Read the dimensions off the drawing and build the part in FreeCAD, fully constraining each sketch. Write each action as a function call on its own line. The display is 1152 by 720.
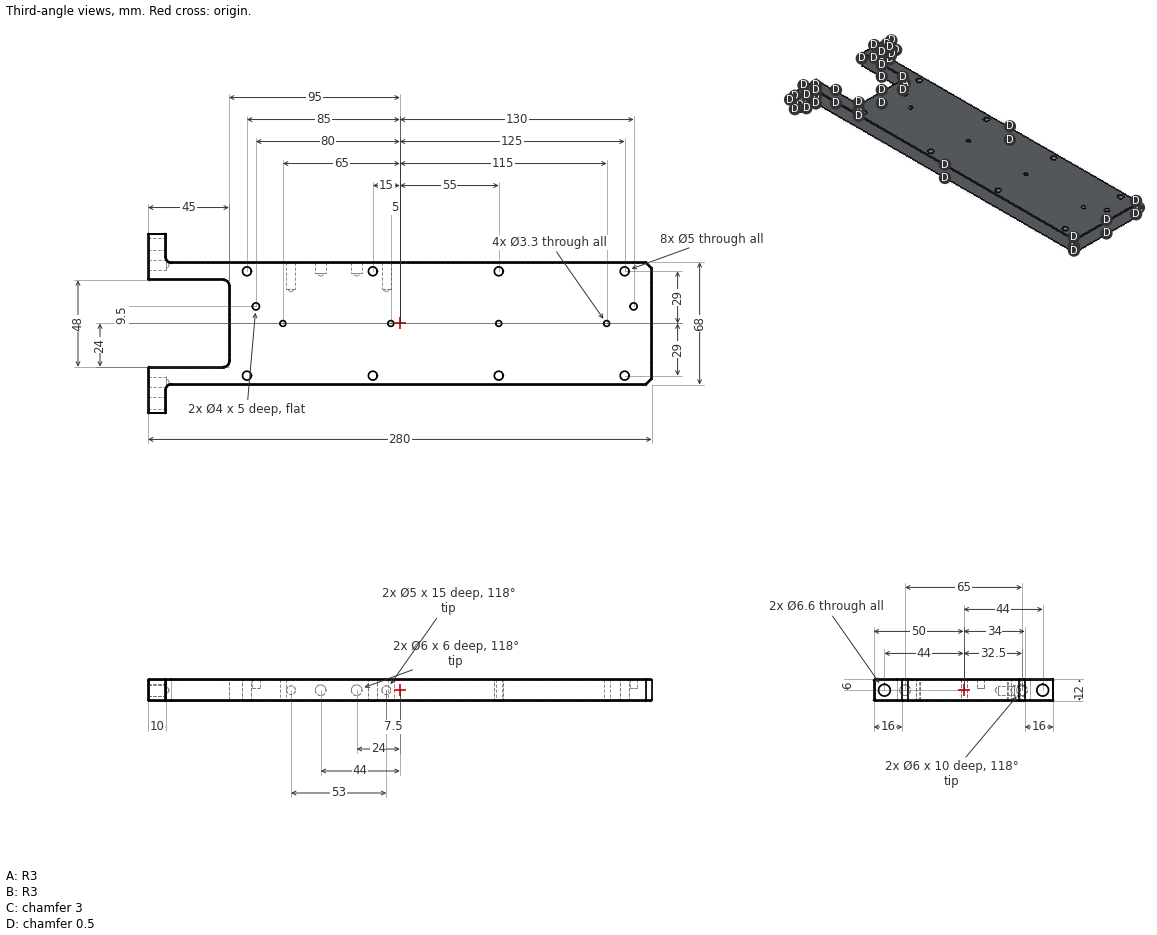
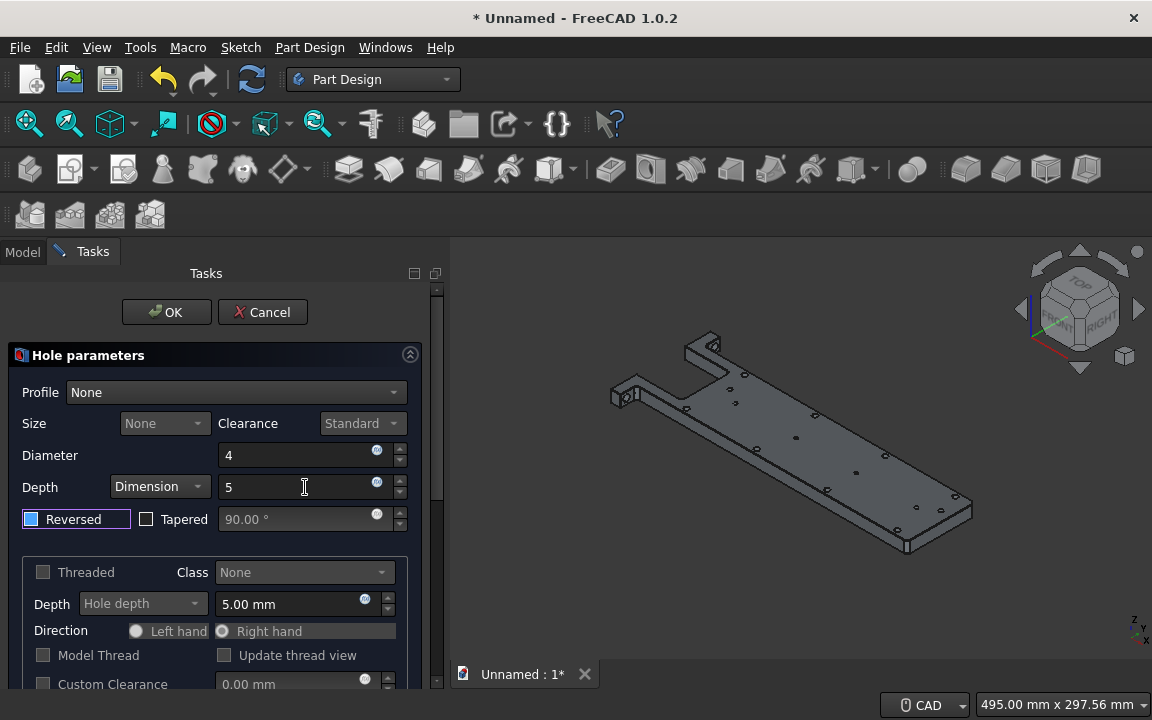
scroll(437, 486, down, 6)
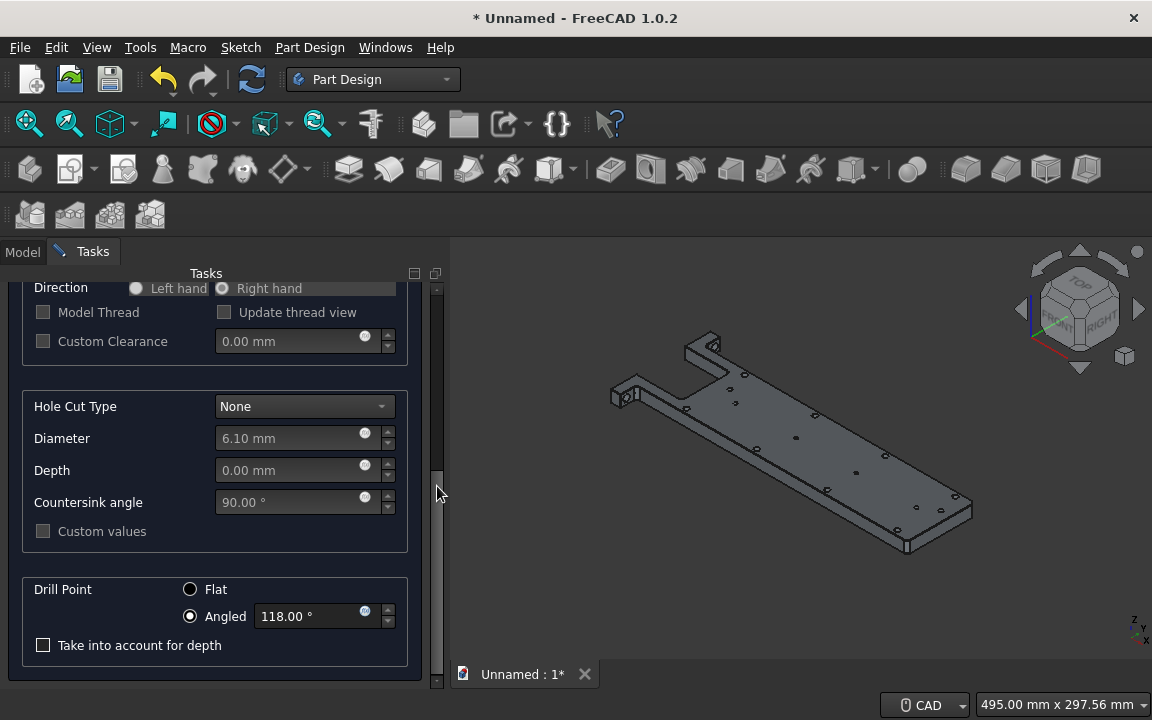
click(191, 589)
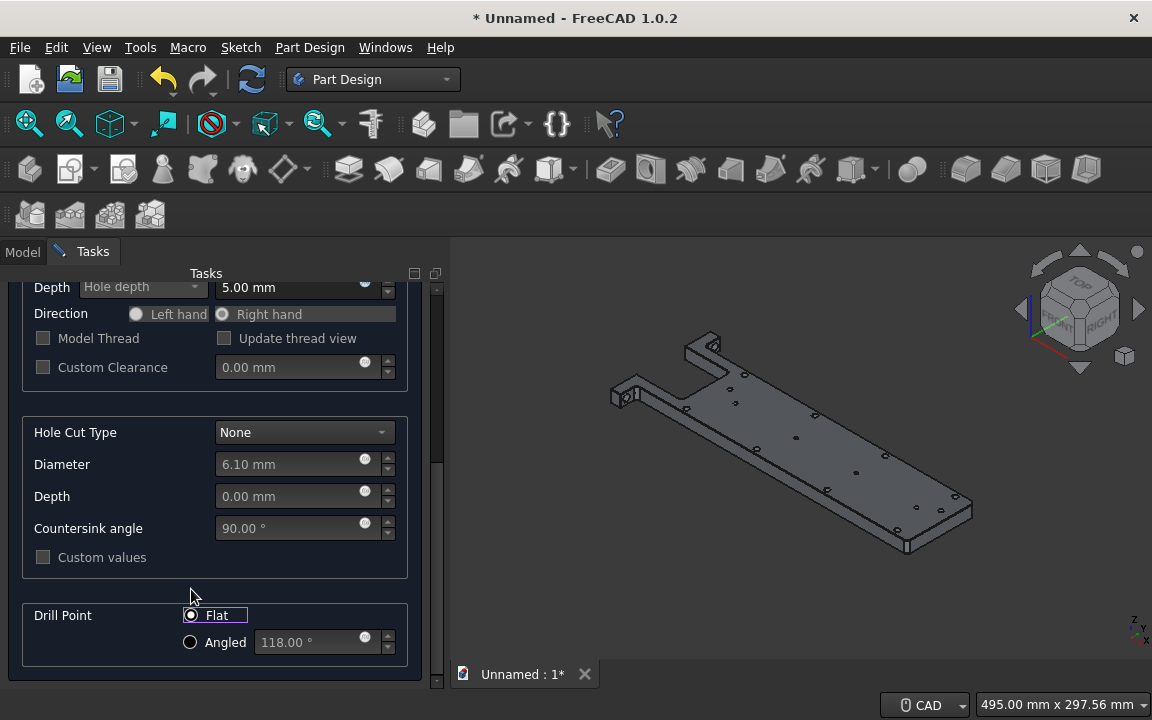
scroll(437, 486, up, 7)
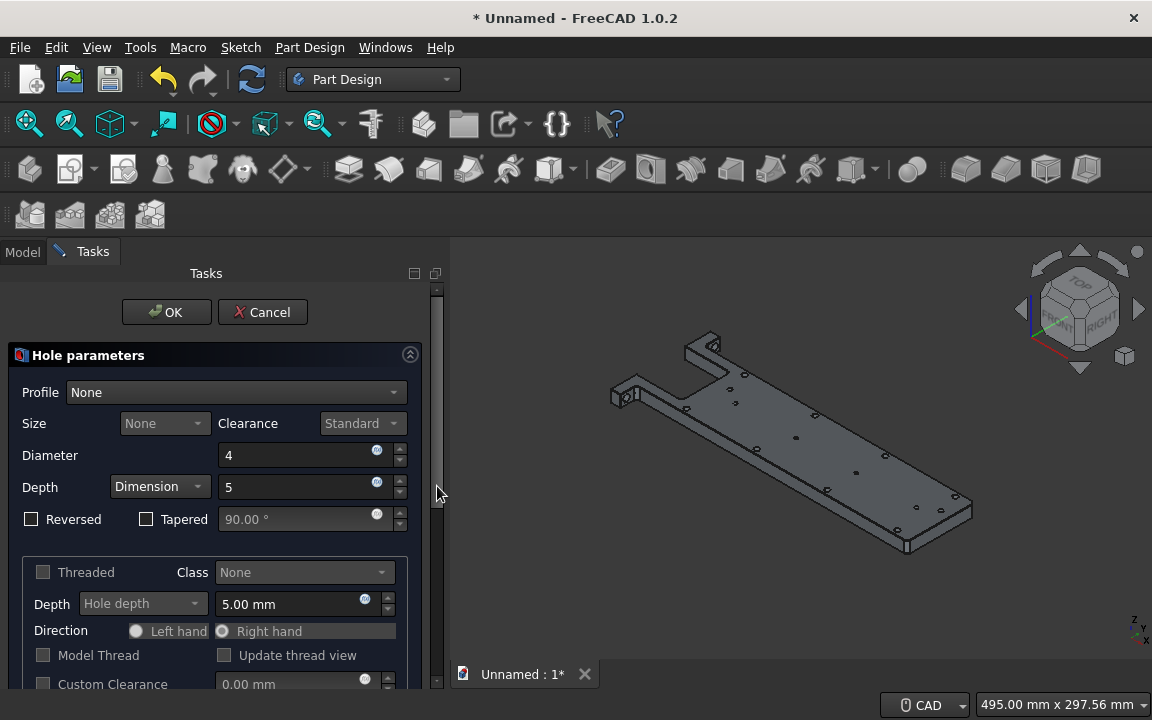
click(167, 312)